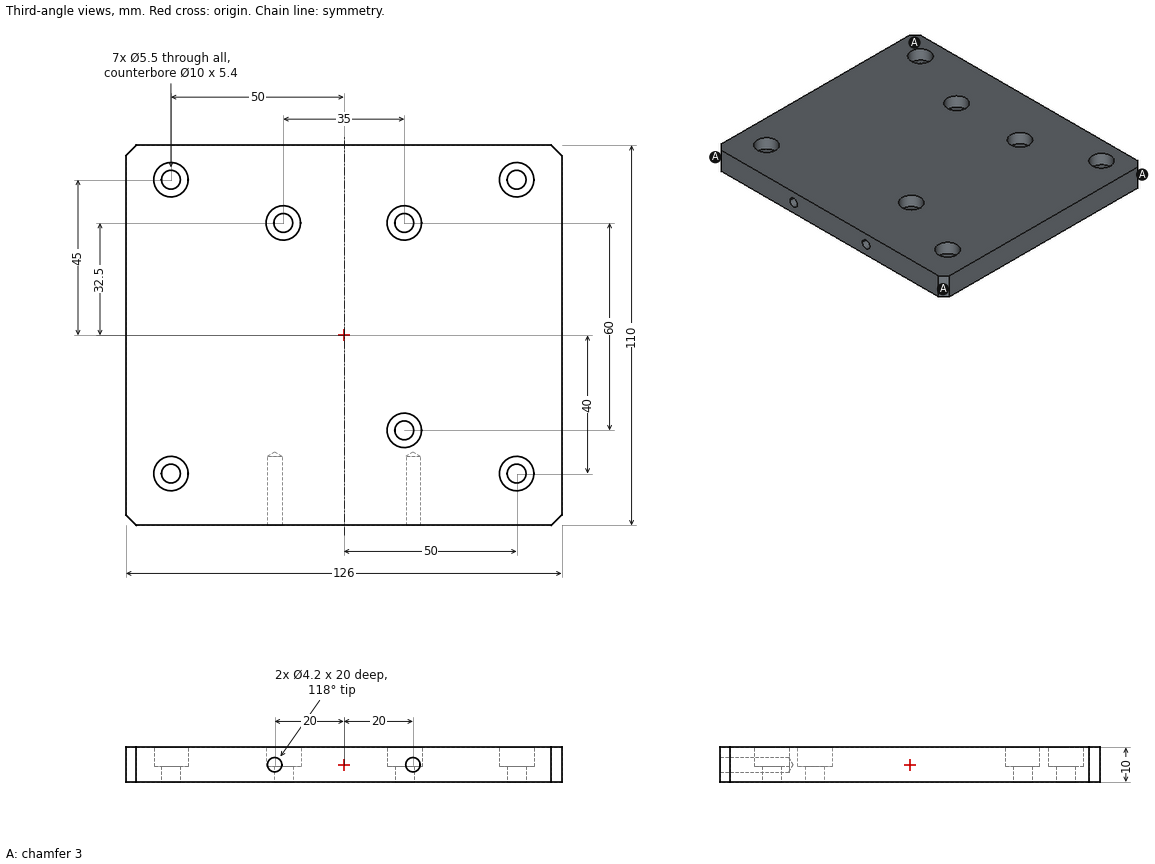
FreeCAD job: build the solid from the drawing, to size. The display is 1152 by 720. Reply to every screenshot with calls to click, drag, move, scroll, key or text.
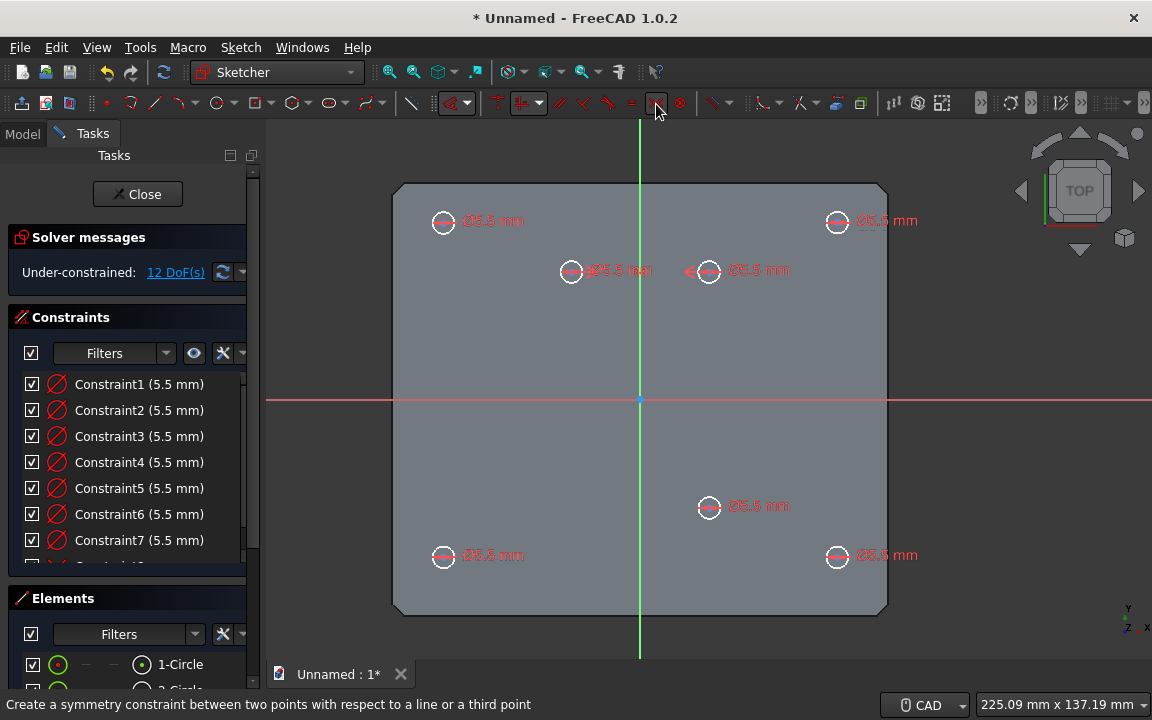
click(444, 223)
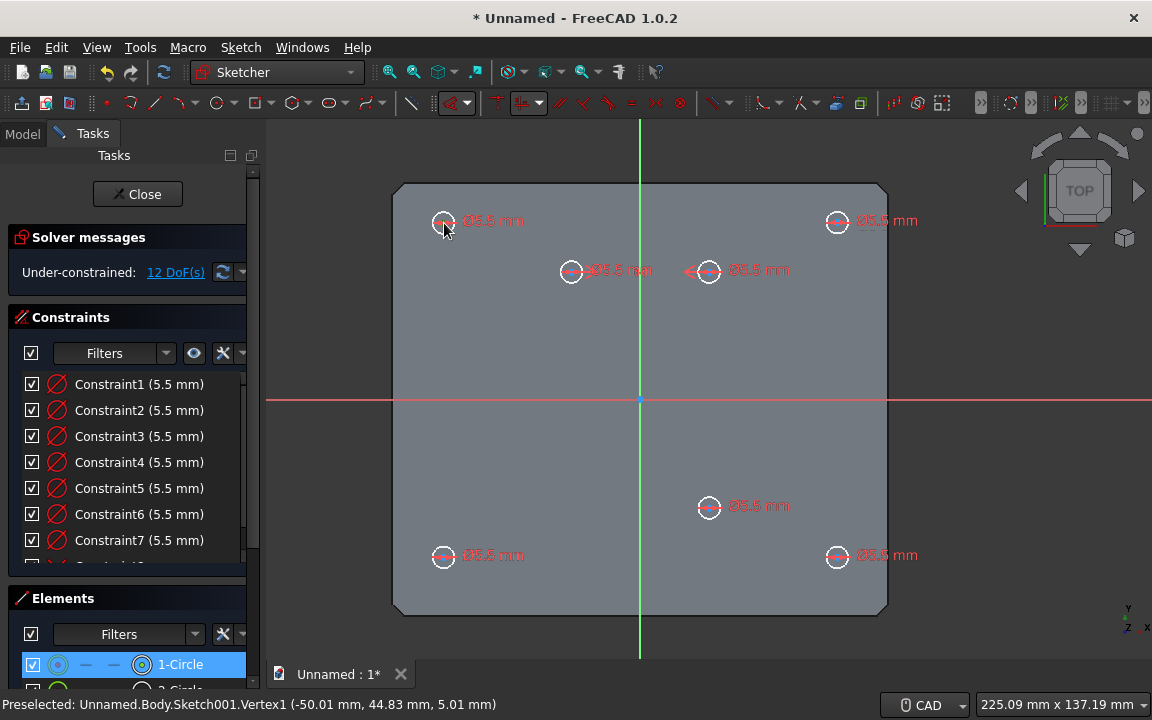
click(837, 223)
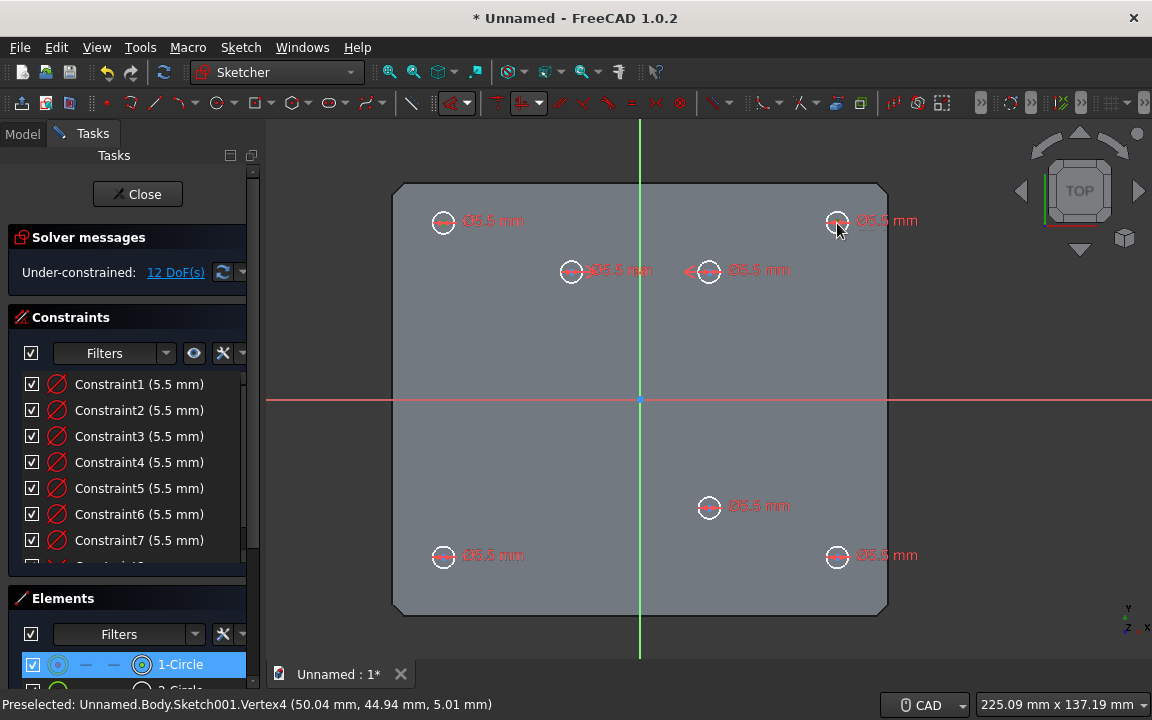
click(640, 596)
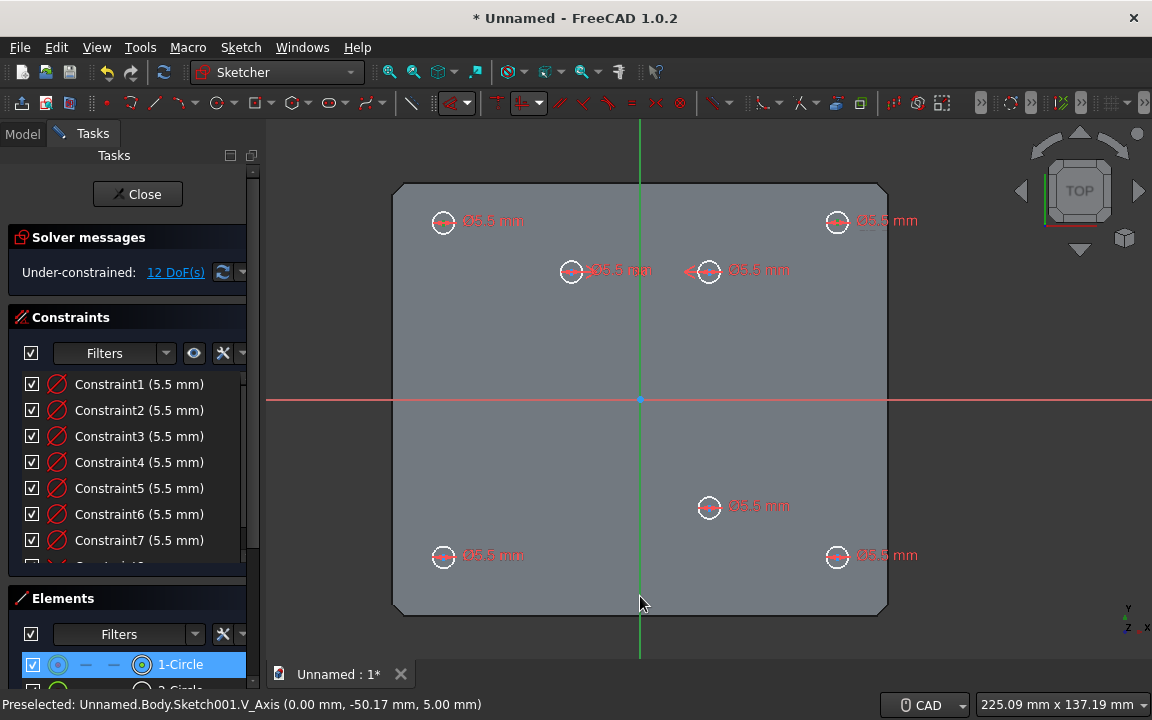
click(656, 104)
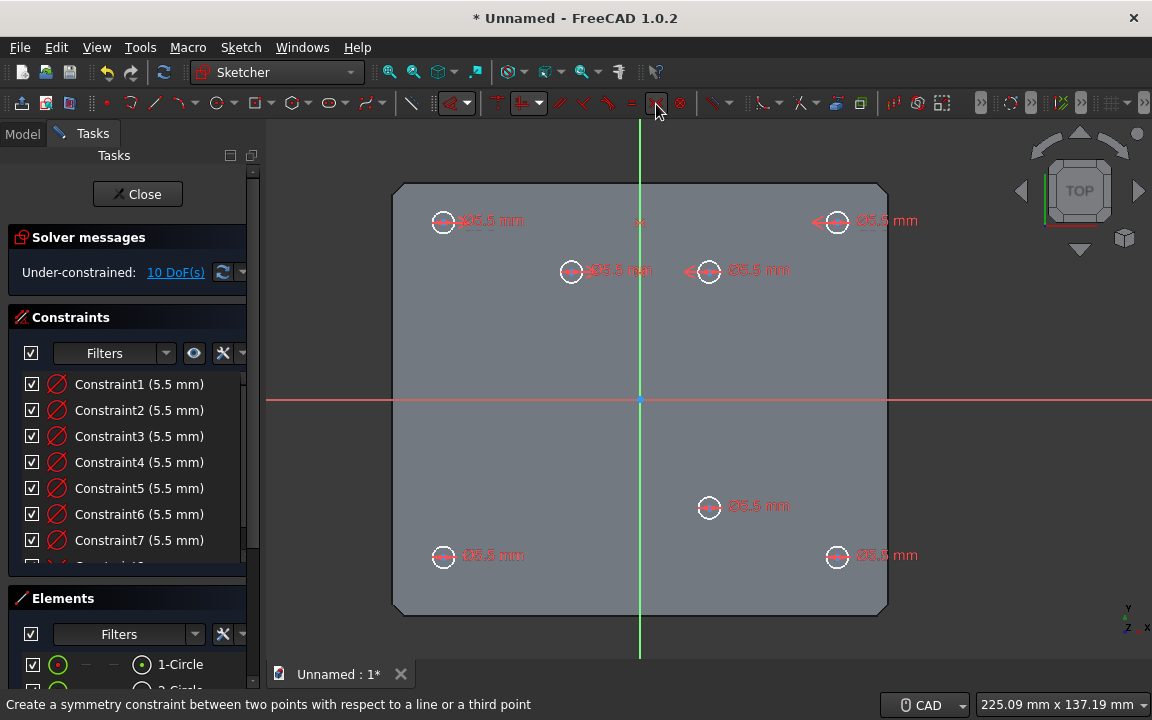
click(837, 557)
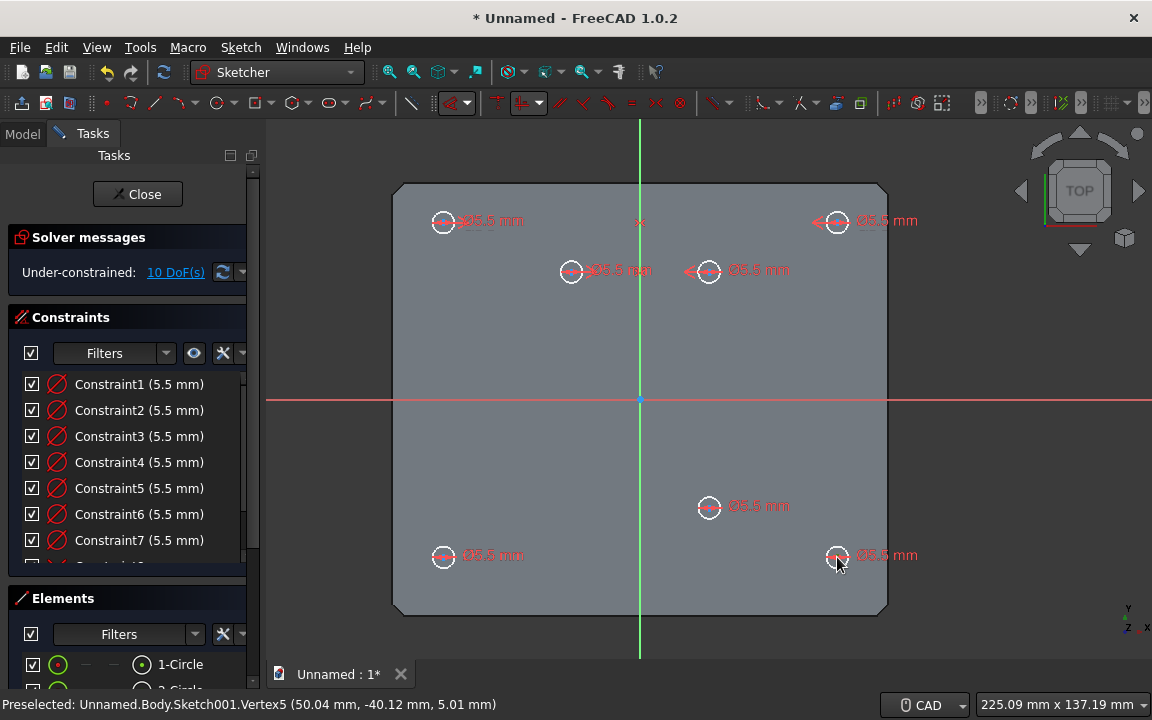
click(444, 557)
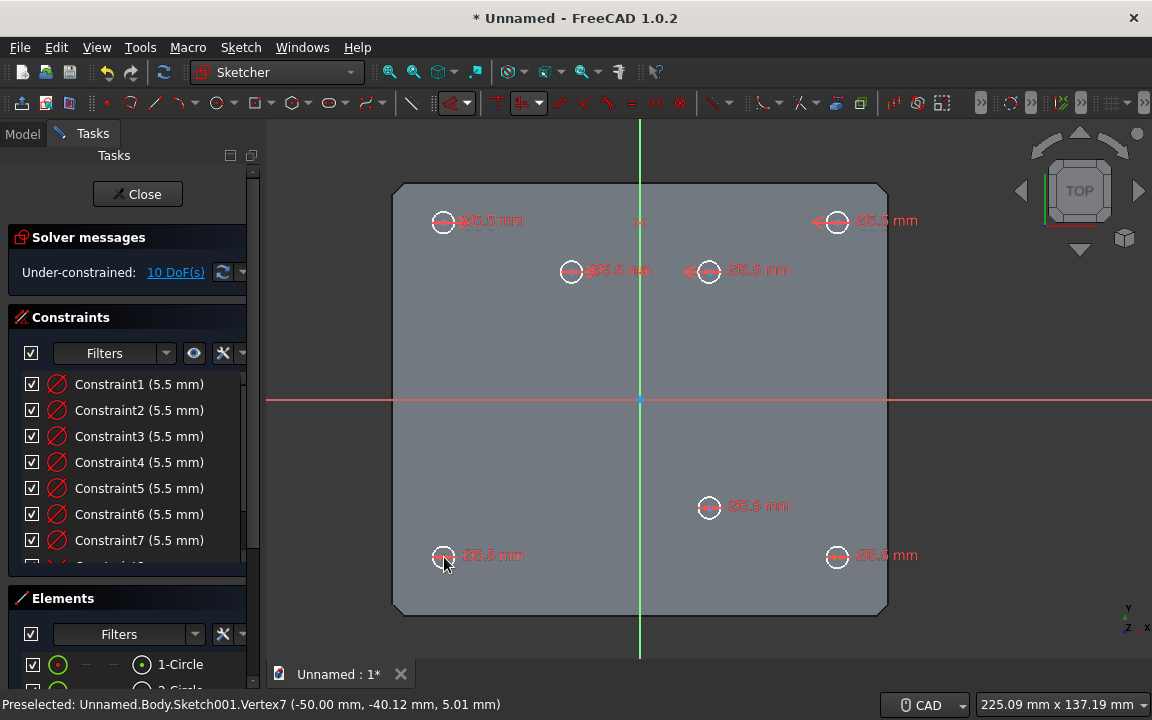
click(640, 596)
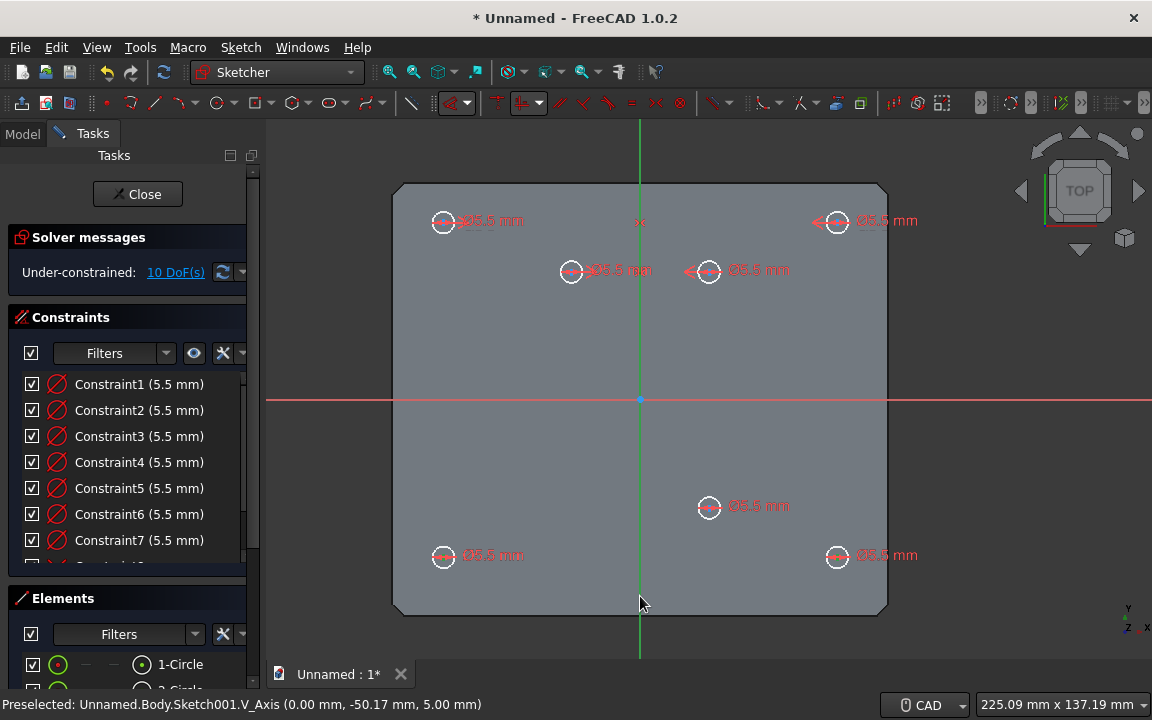
click(656, 104)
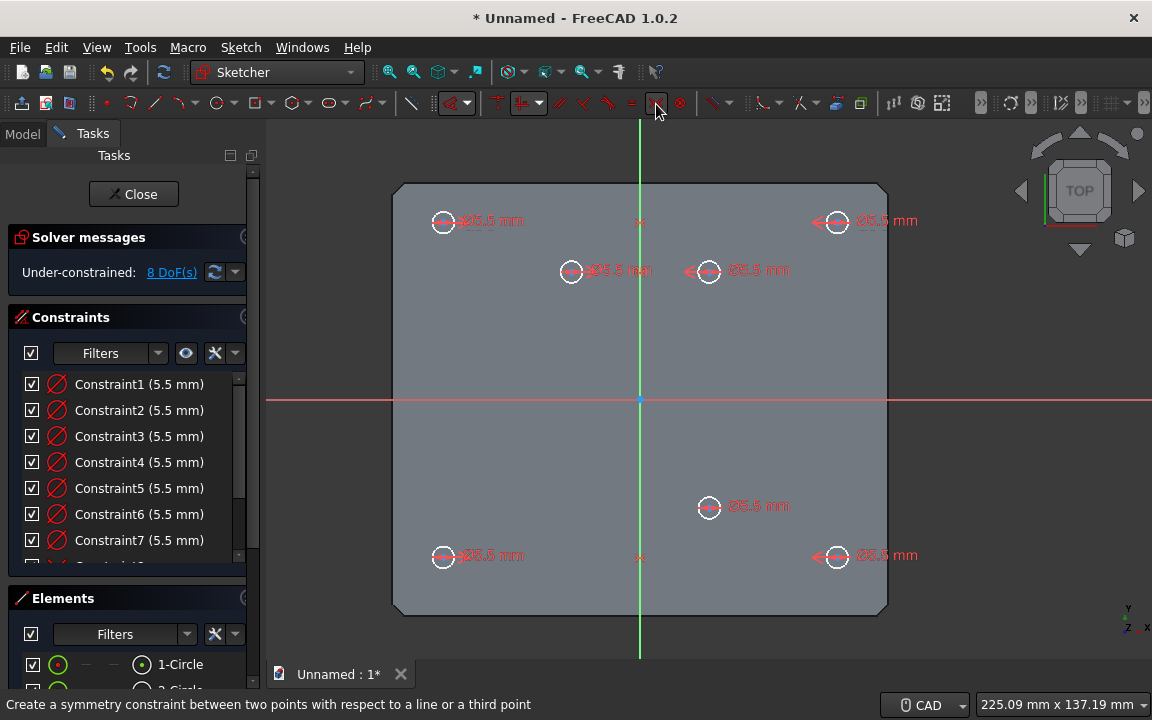
click(450, 104)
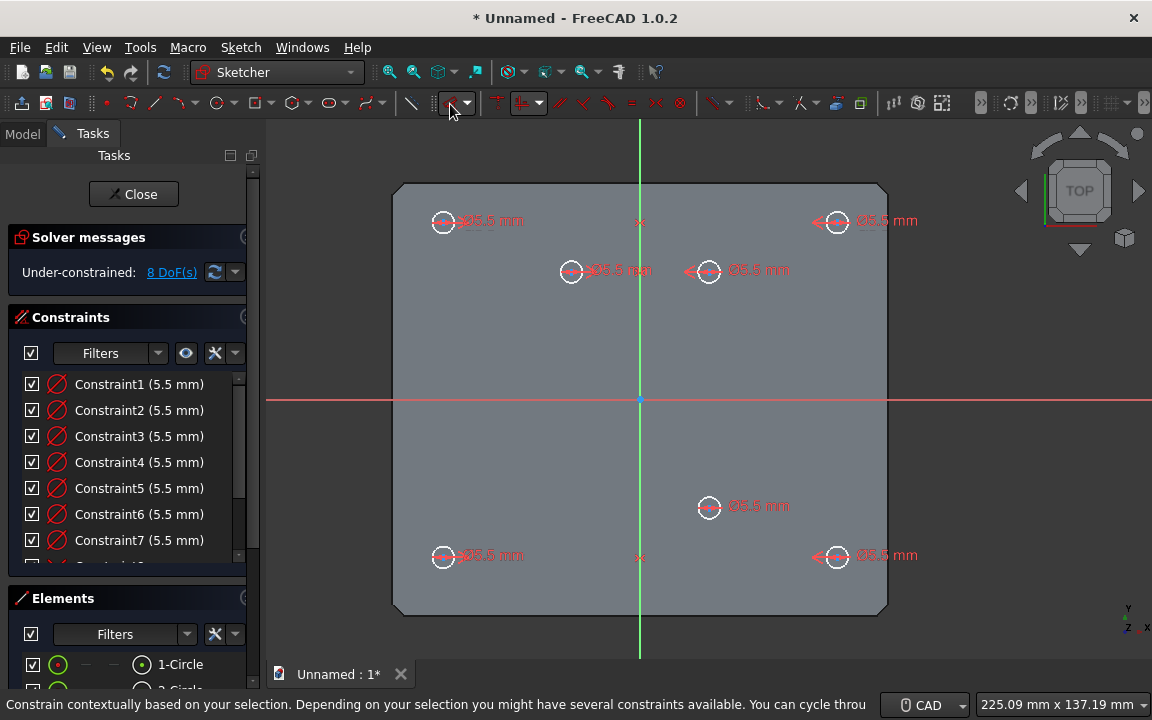
click(443, 223)
click(542, 189)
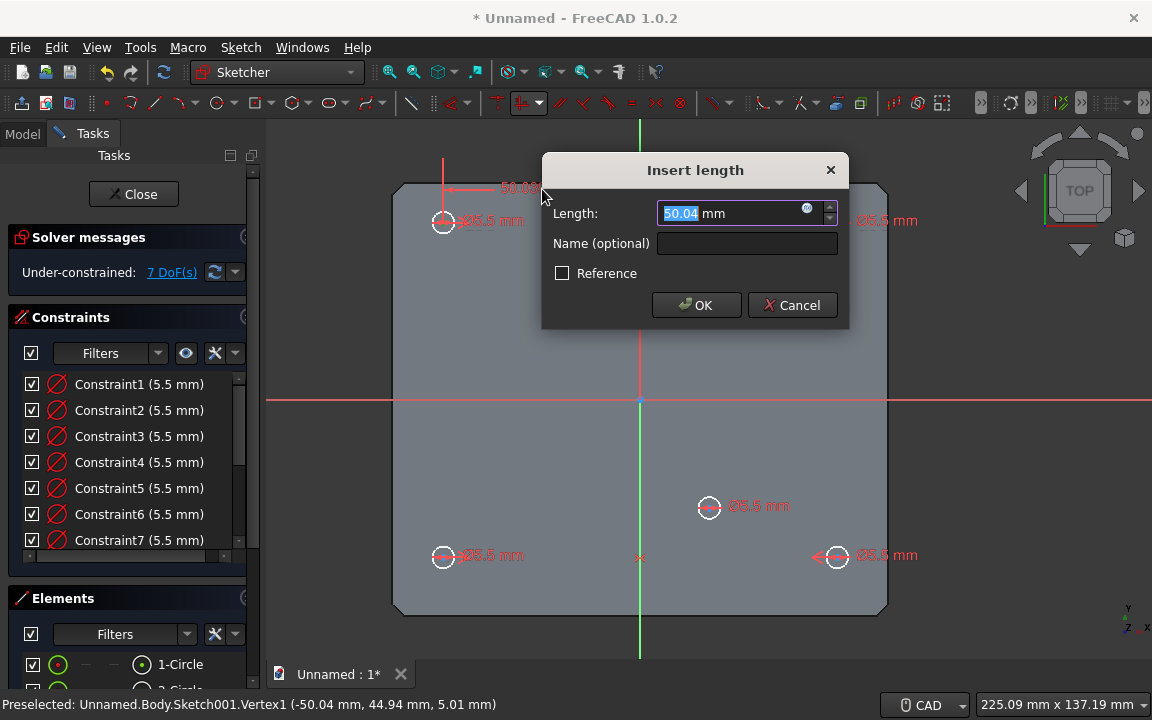
text(50)
key(Return)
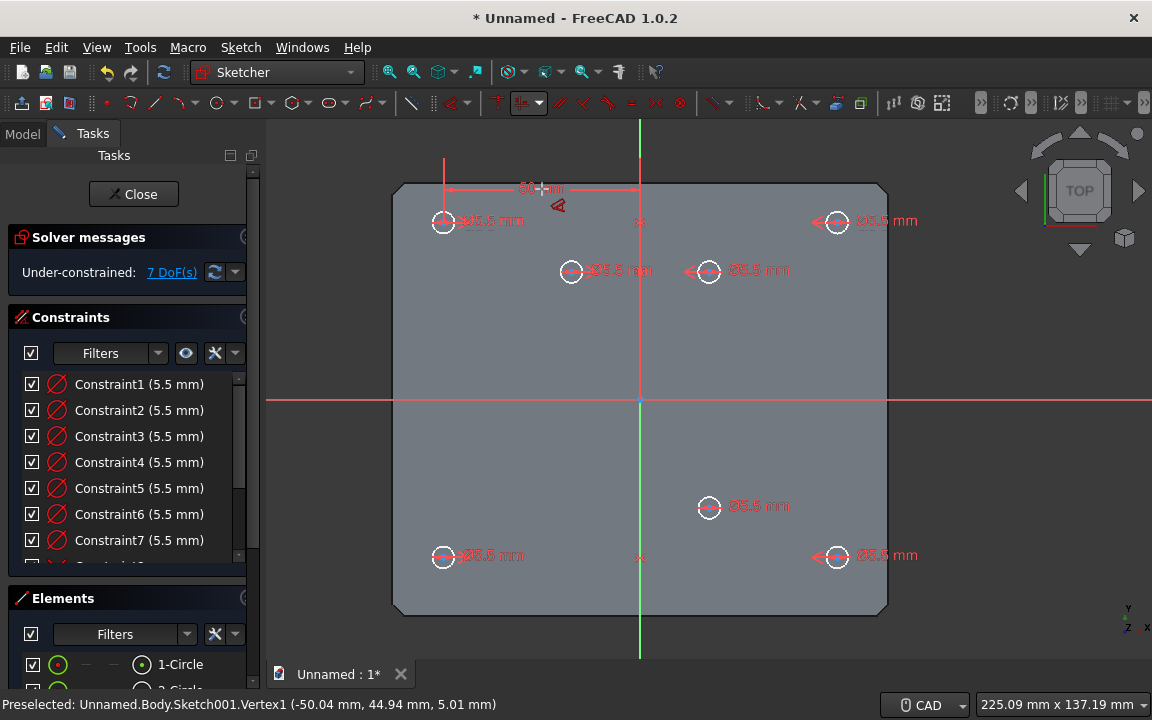
click(444, 223)
click(410, 311)